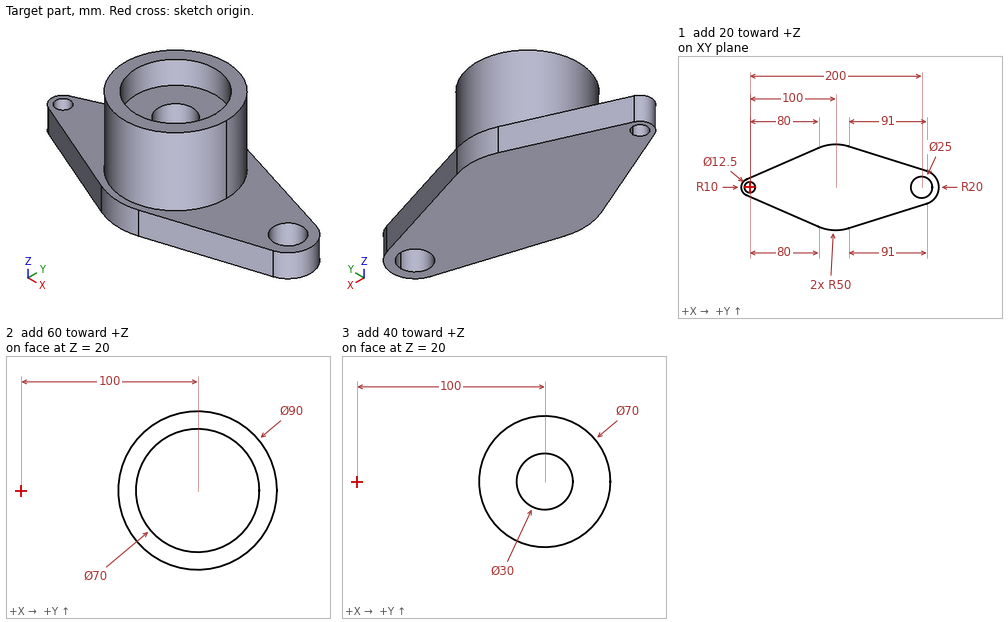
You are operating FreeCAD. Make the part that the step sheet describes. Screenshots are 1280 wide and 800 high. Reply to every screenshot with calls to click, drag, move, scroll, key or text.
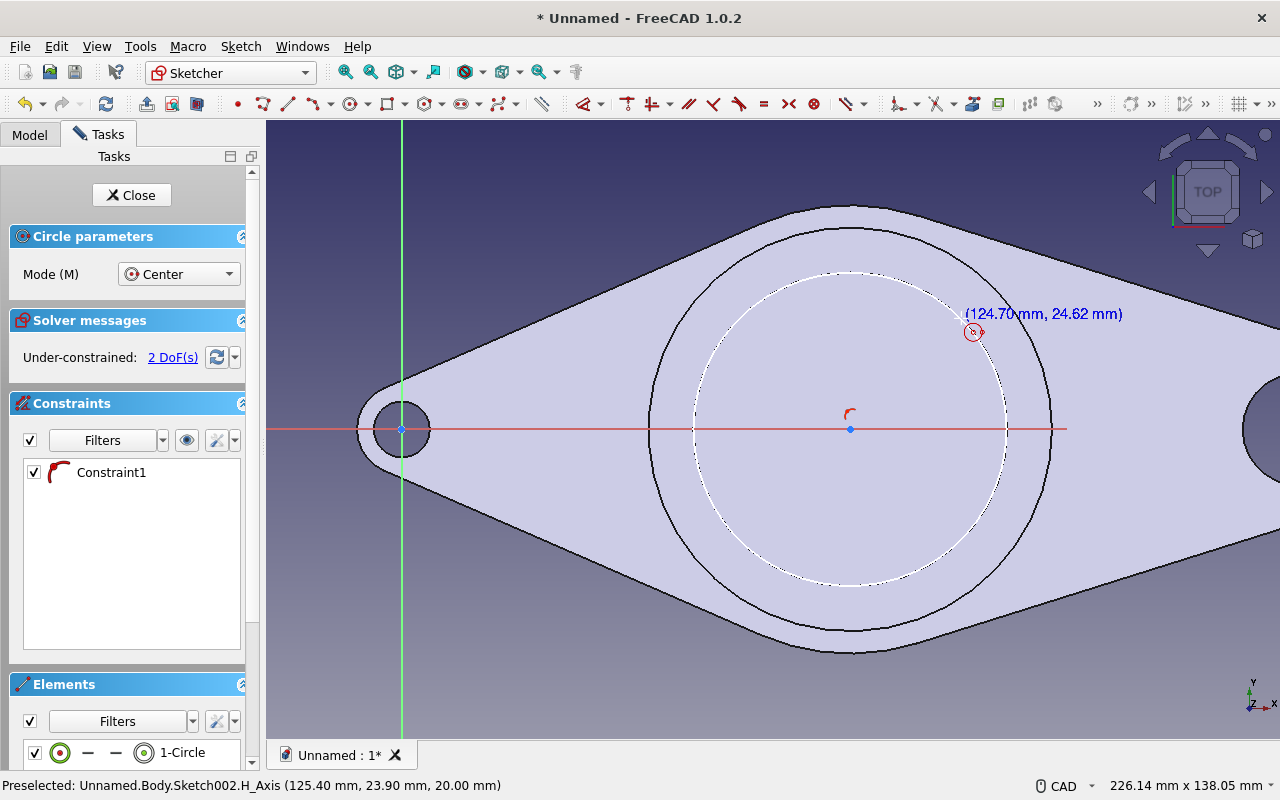
click(850, 429)
click(898, 382)
key(Escape)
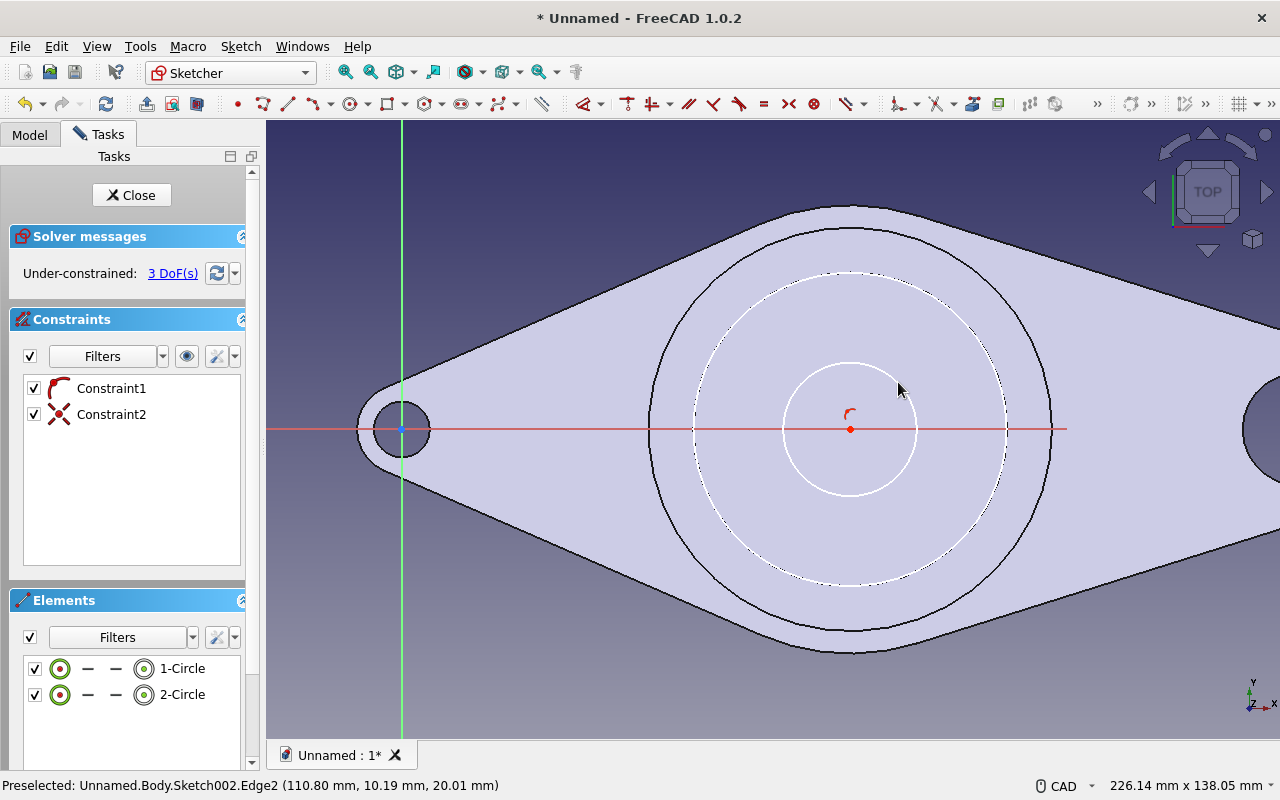
click(582, 104)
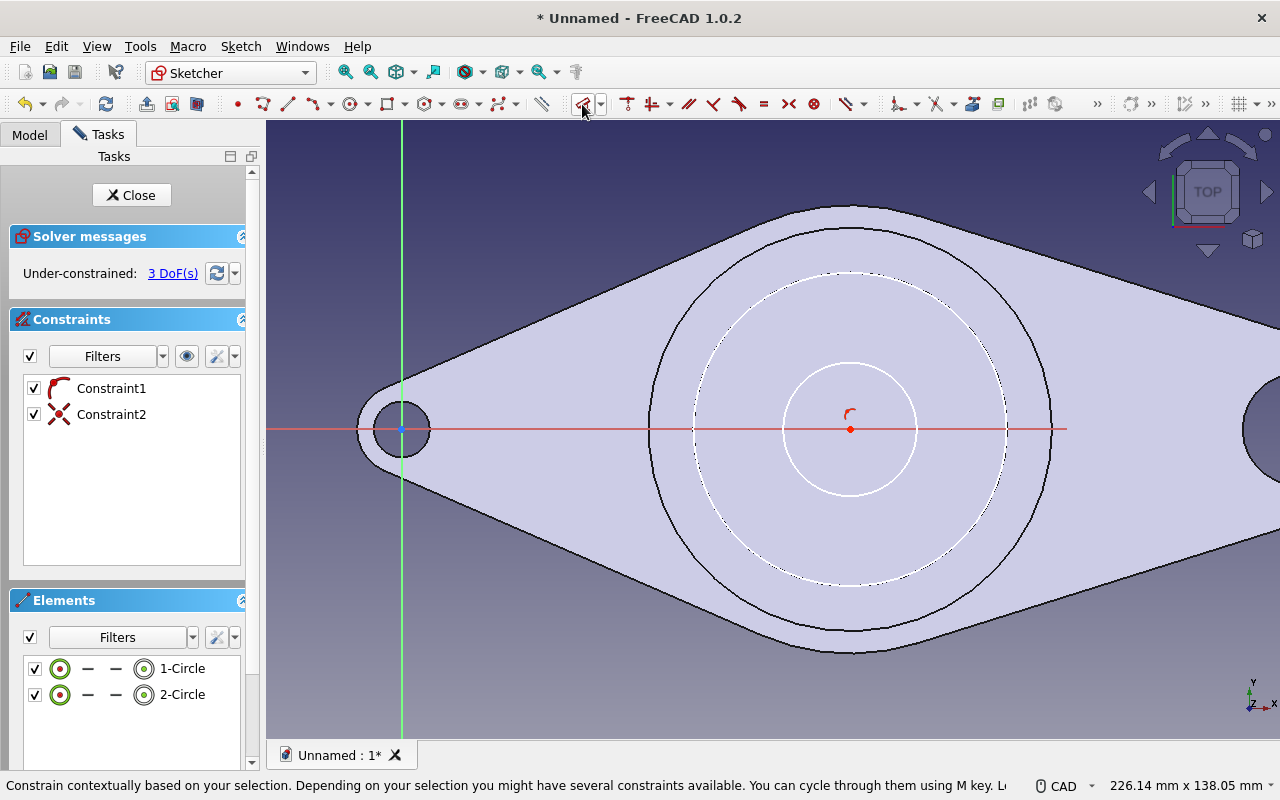
click(960, 318)
click(982, 295)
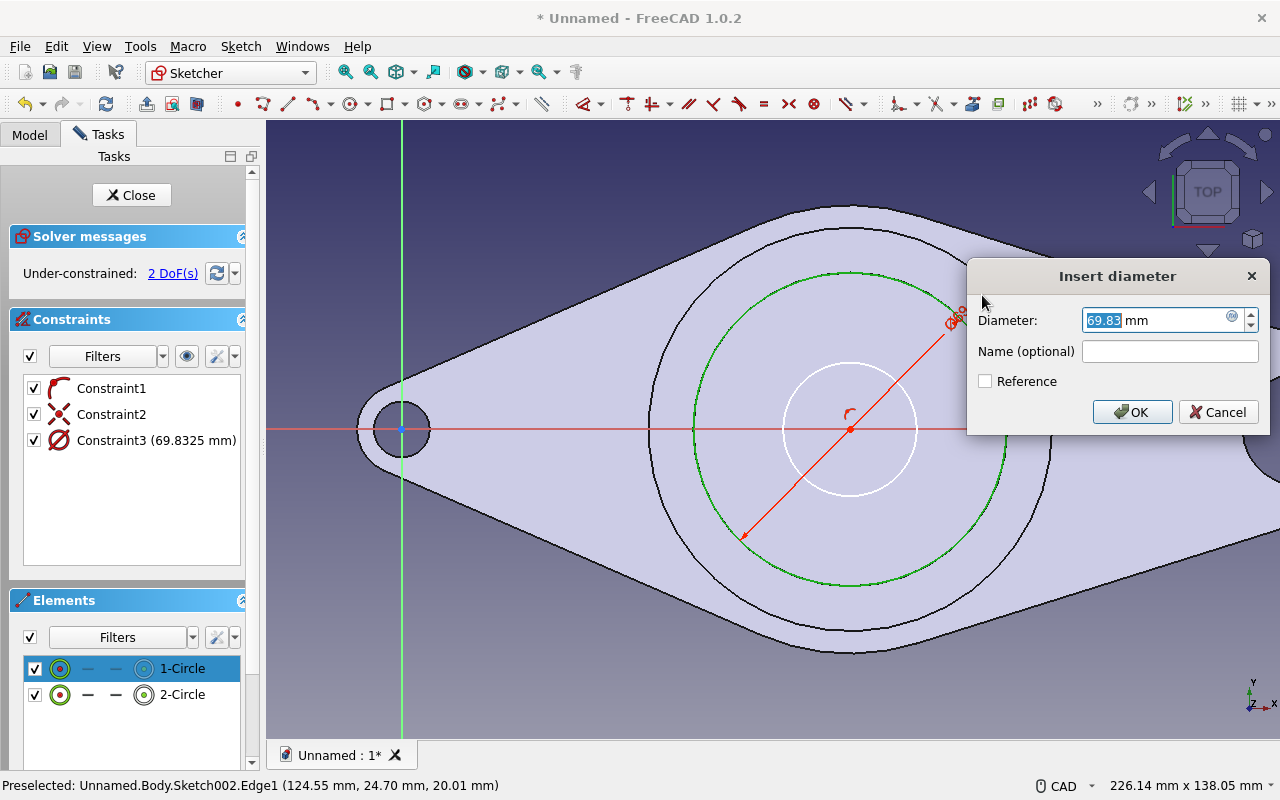
text(70)
key(Return)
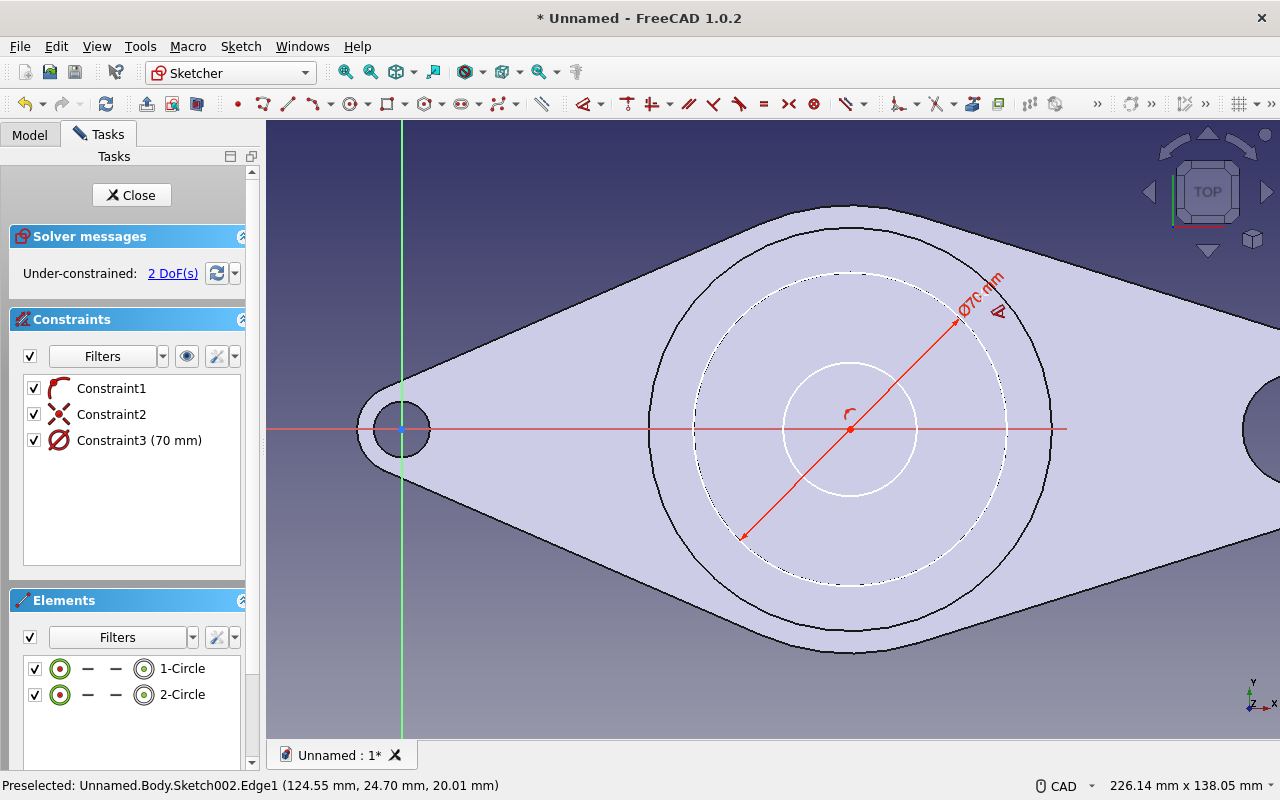
click(897, 382)
click(920, 359)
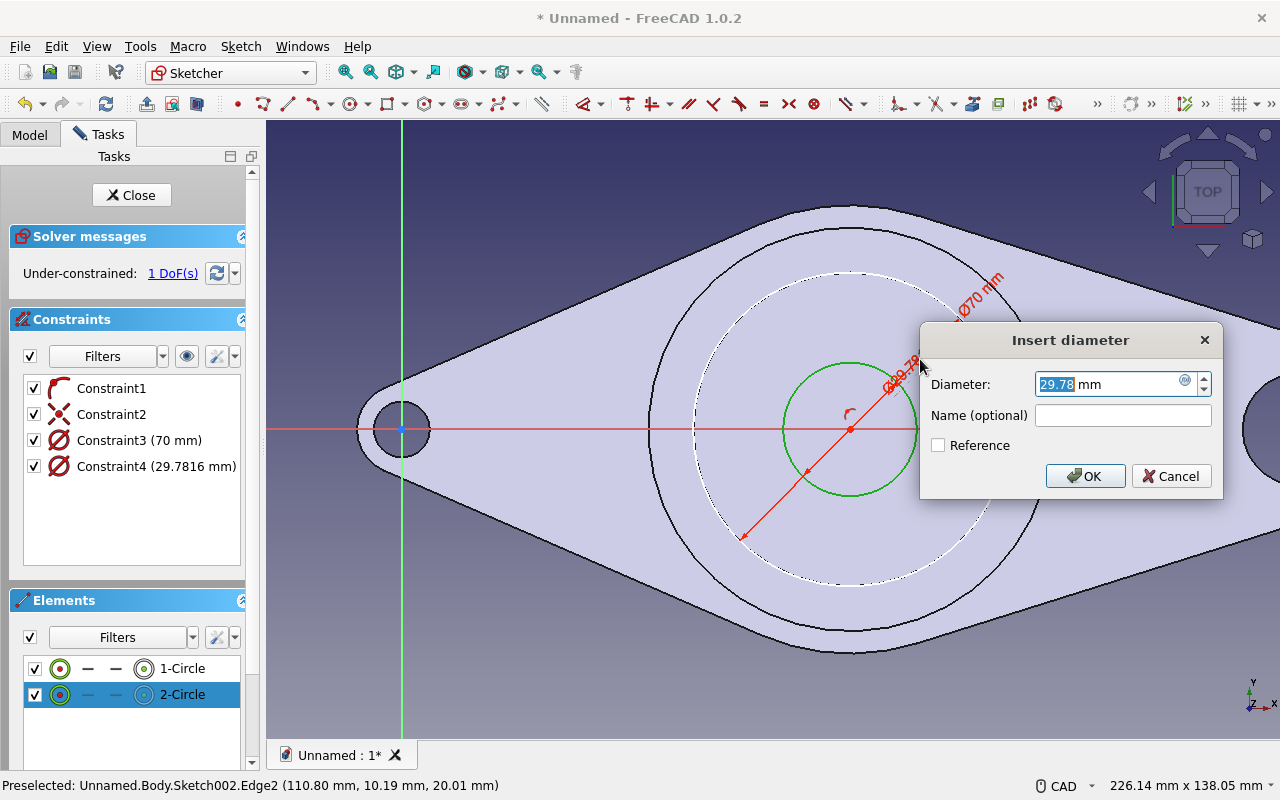
text(30)
key(Return)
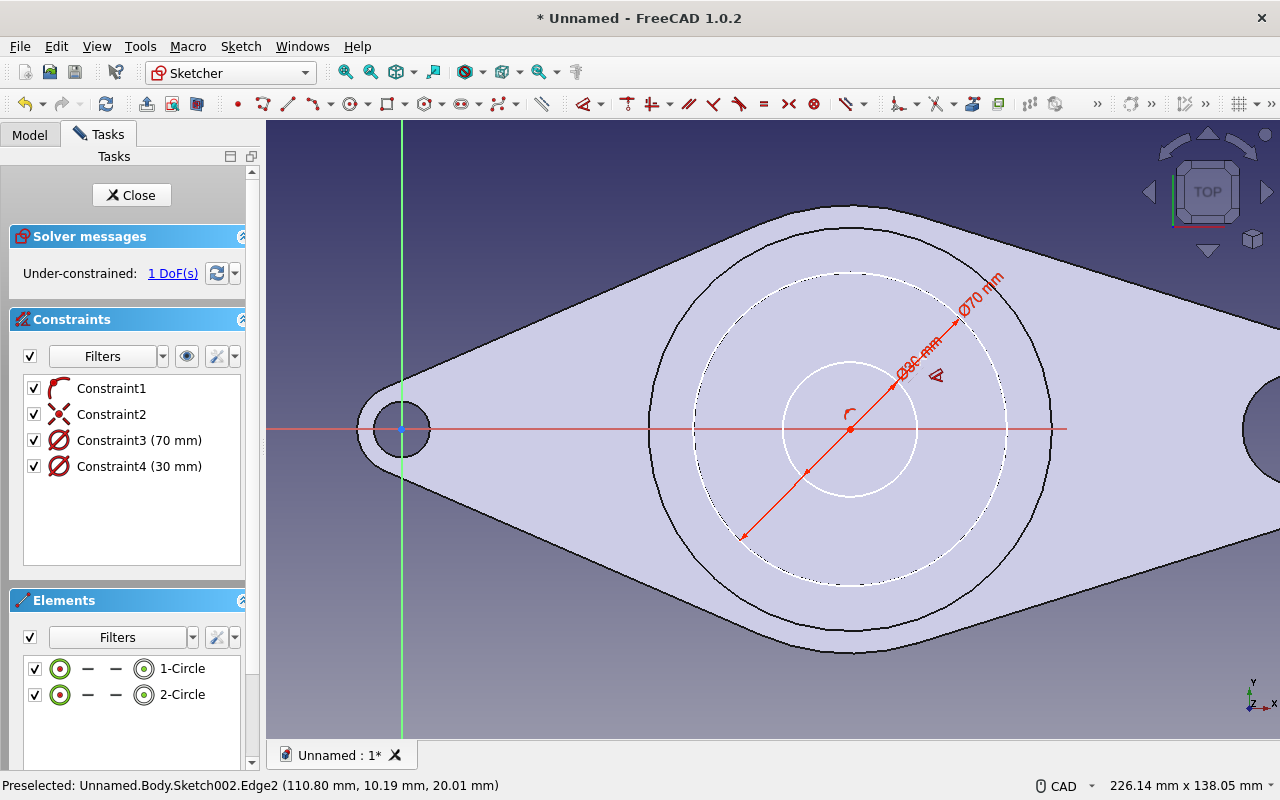
click(850, 429)
click(626, 463)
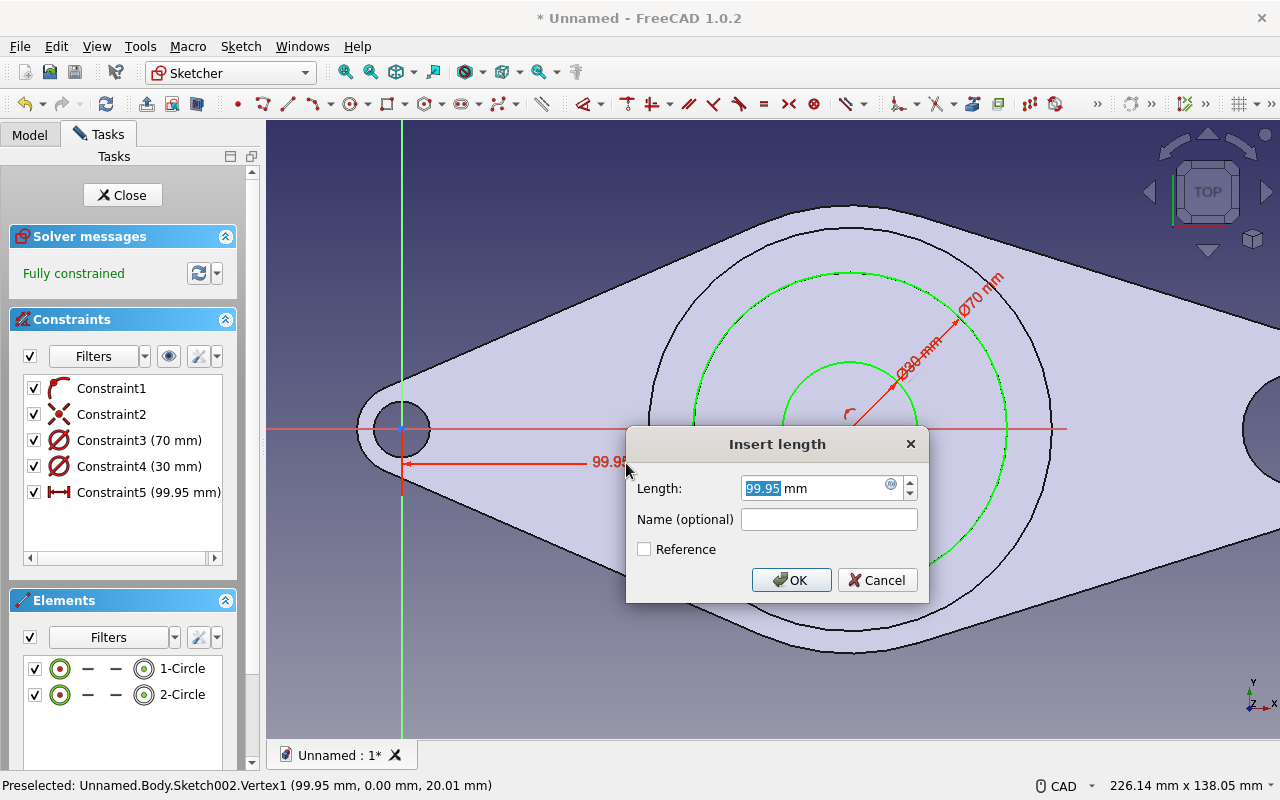
text(100)
key(Return)
key(Escape)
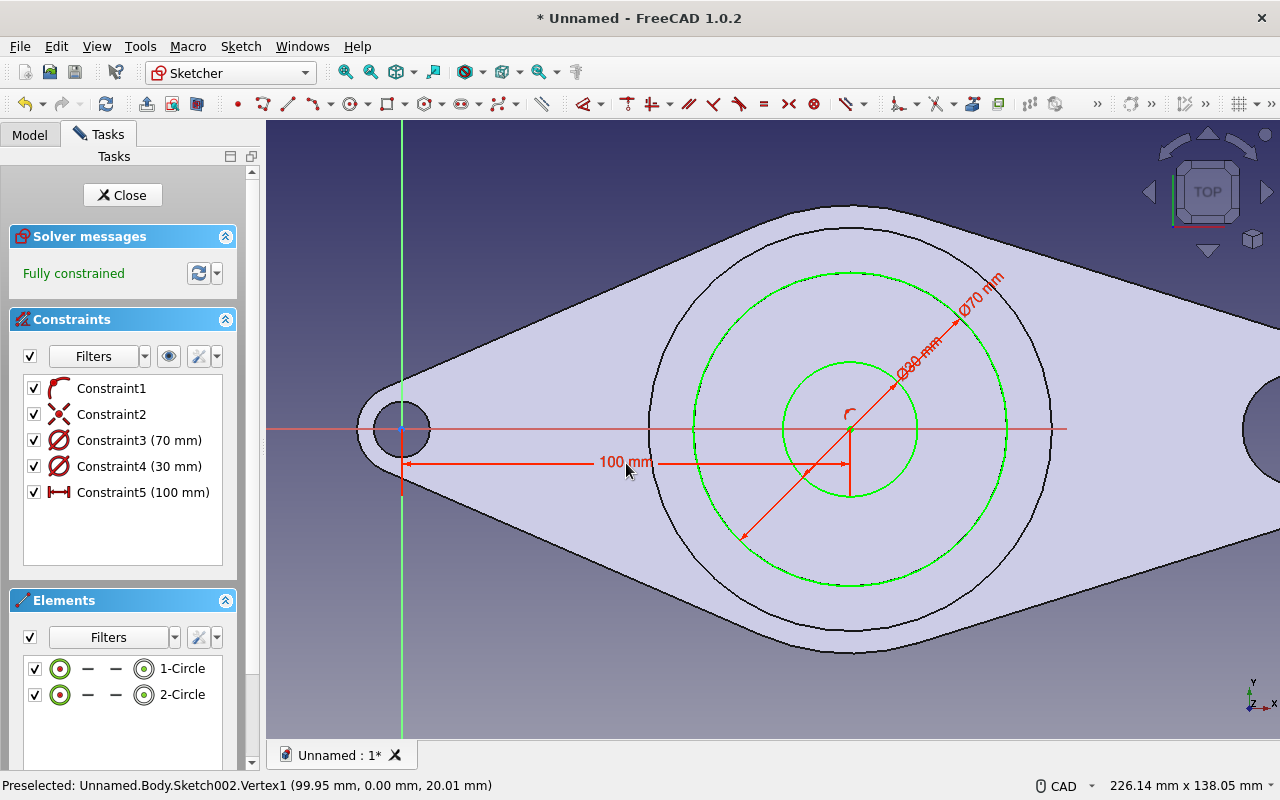
click(123, 195)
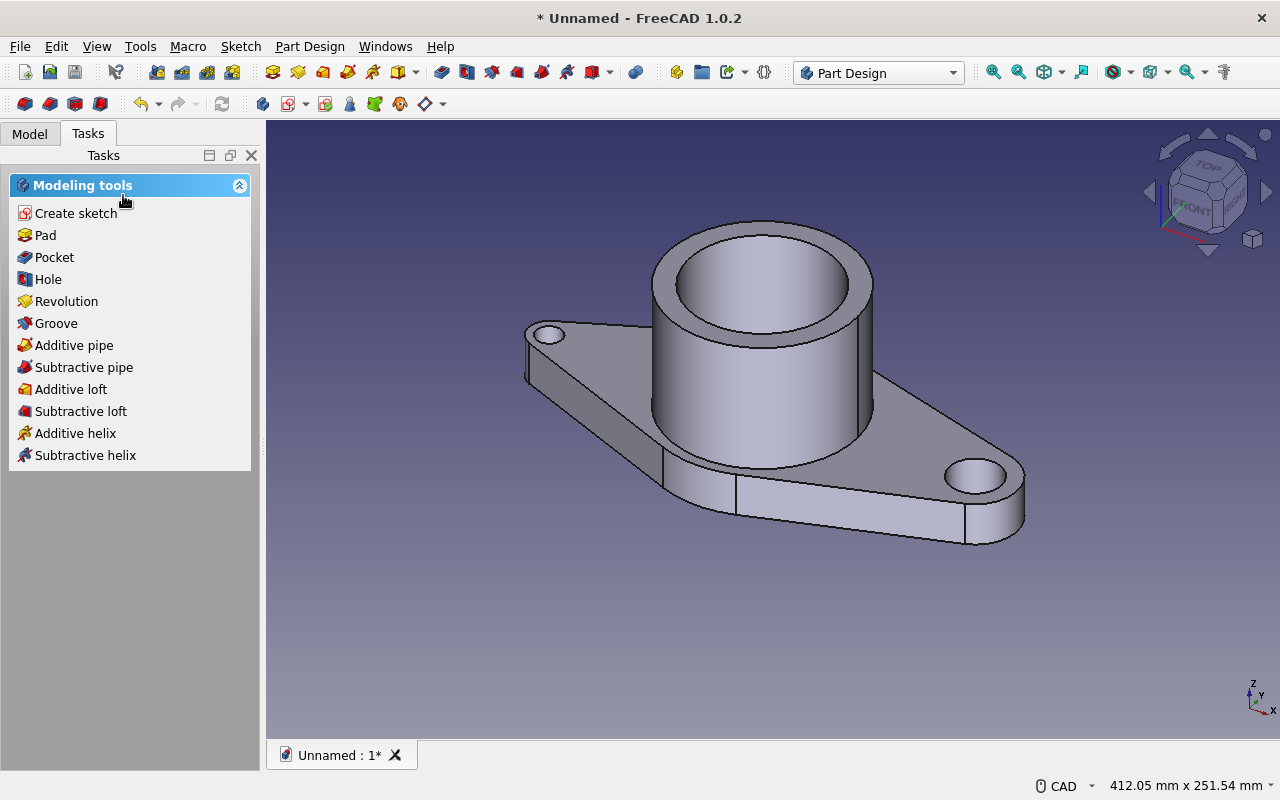
click(273, 72)